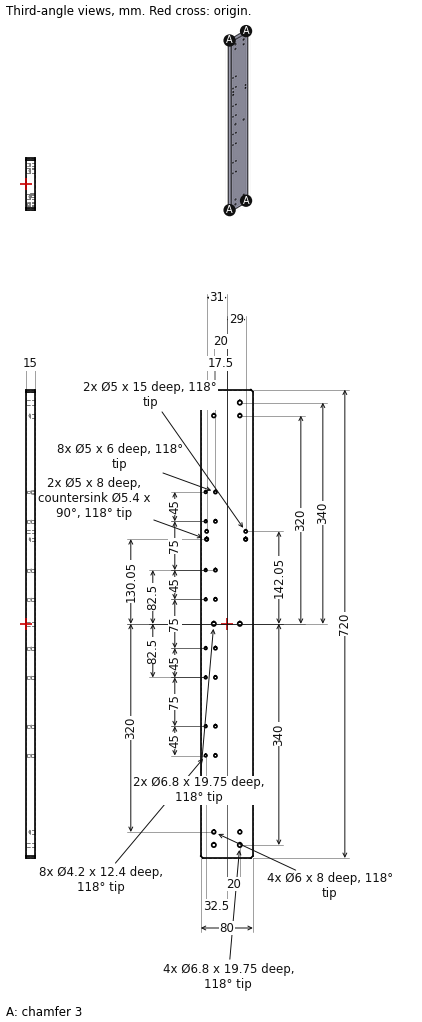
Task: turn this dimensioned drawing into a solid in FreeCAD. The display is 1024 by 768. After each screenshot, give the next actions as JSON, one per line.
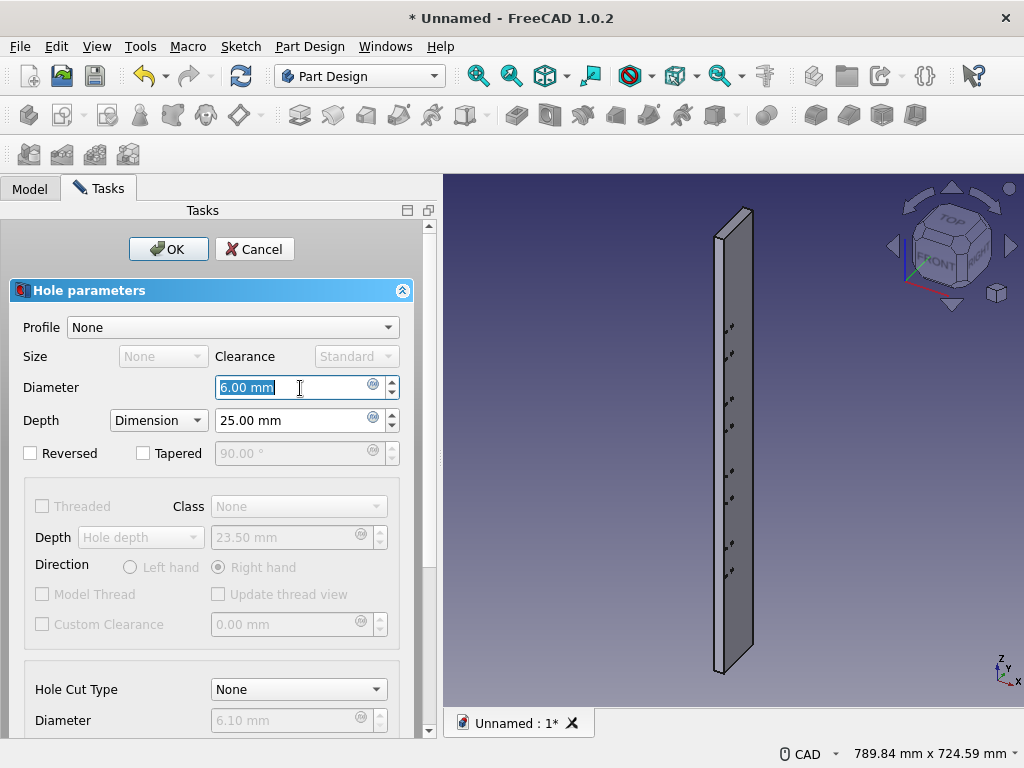
{"action": "type", "text": "5"}
{"action": "key", "text": "Tab"}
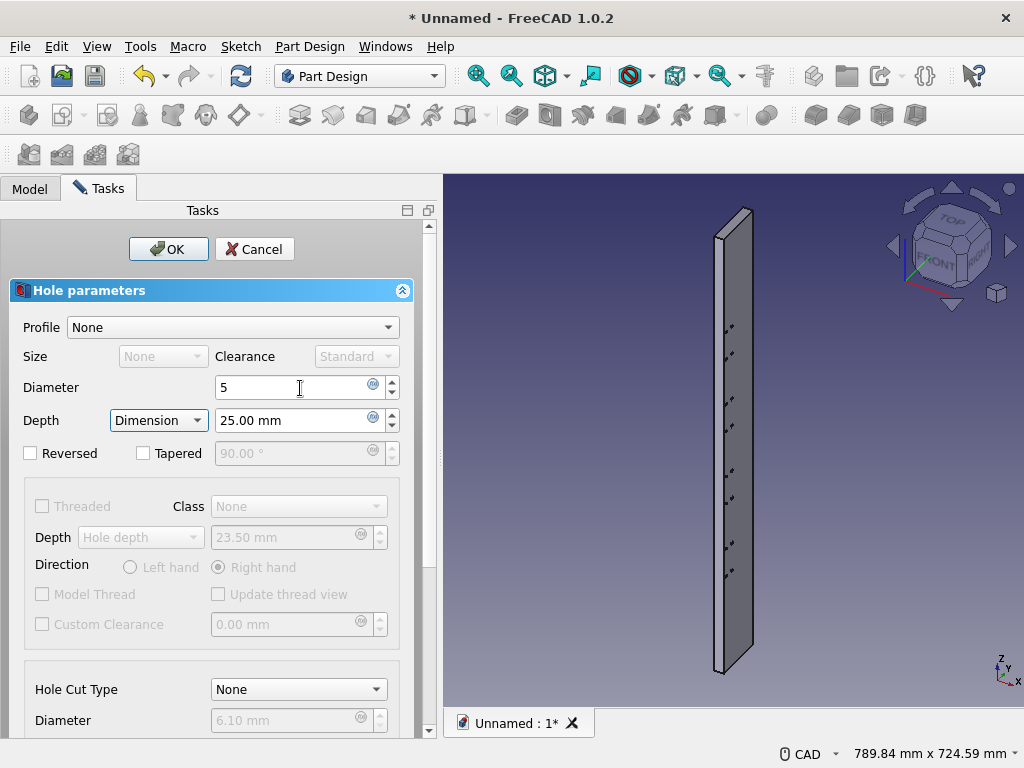
{"action": "triple_click", "coordinate": [300, 420]}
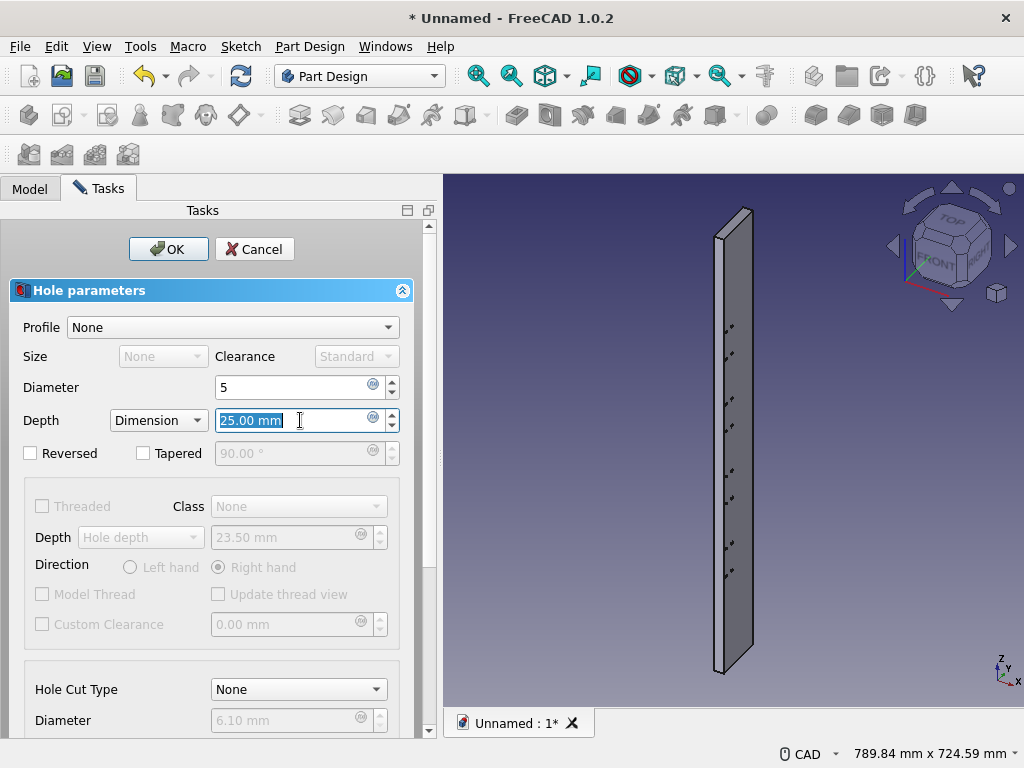
{"action": "type", "text": "6"}
{"action": "key", "text": "Tab"}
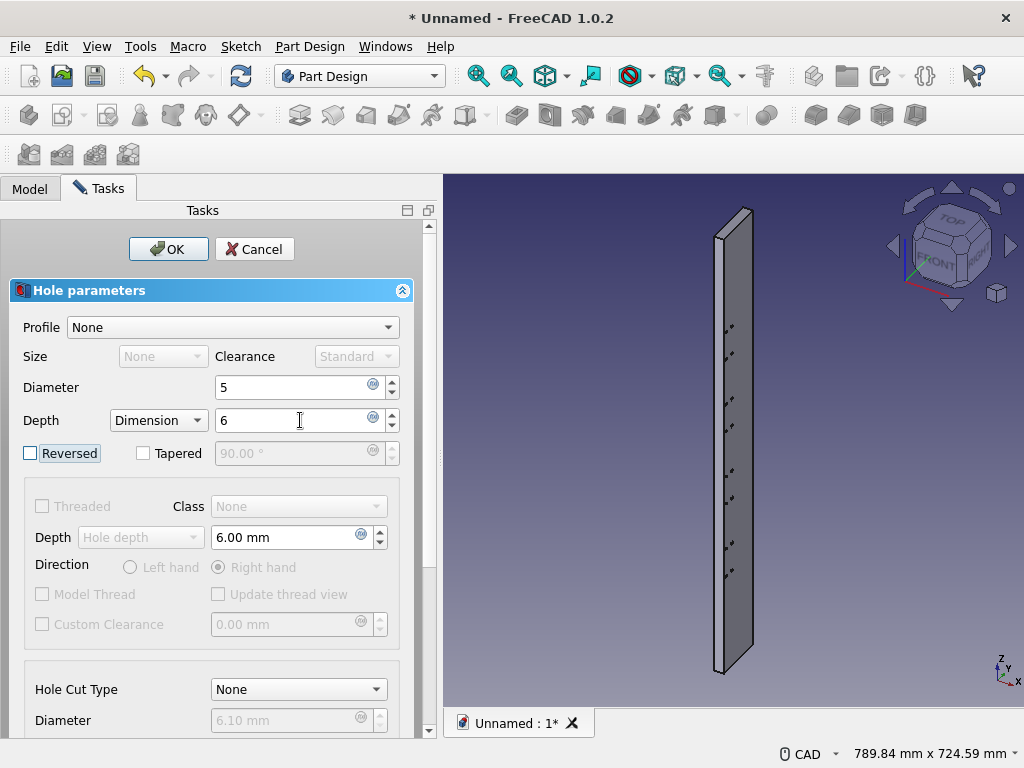
{"action": "left_click", "coordinate": [169, 249]}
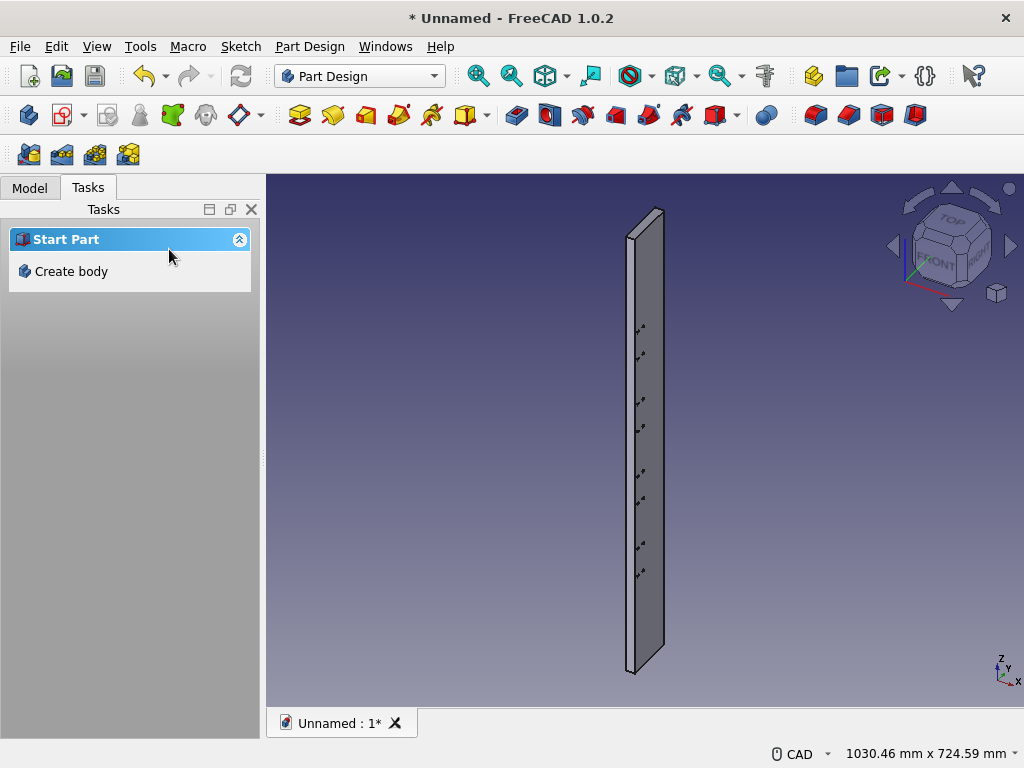
{"action": "left_click", "coordinate": [650, 627]}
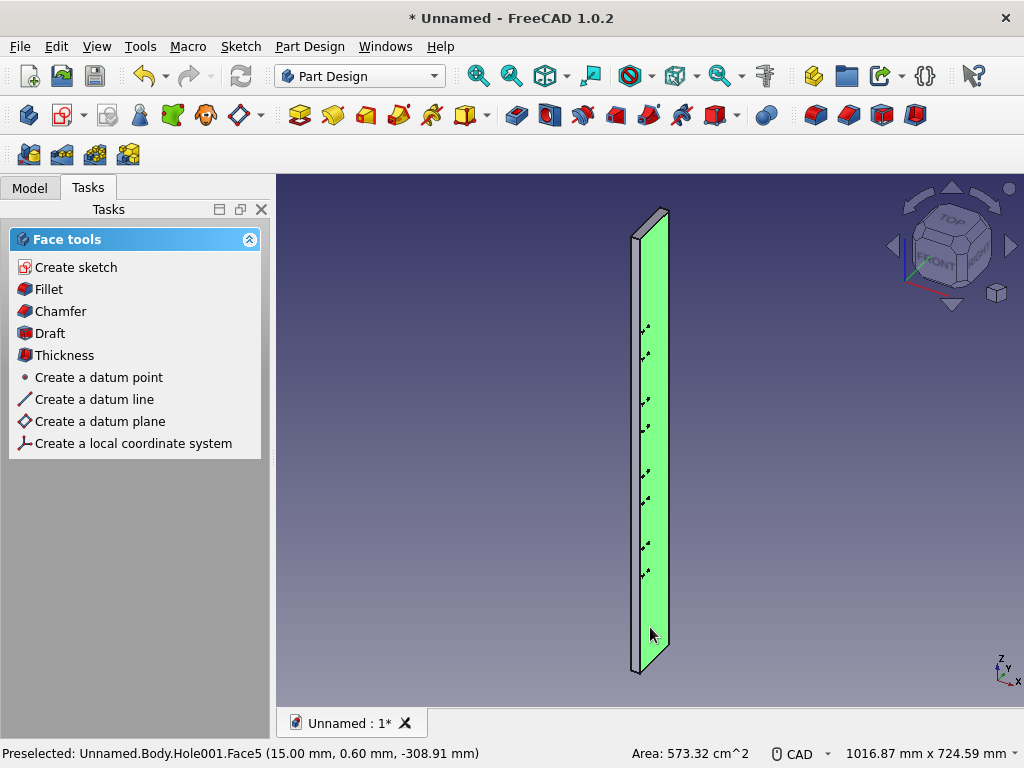
{"action": "left_click", "coordinate": [62, 116]}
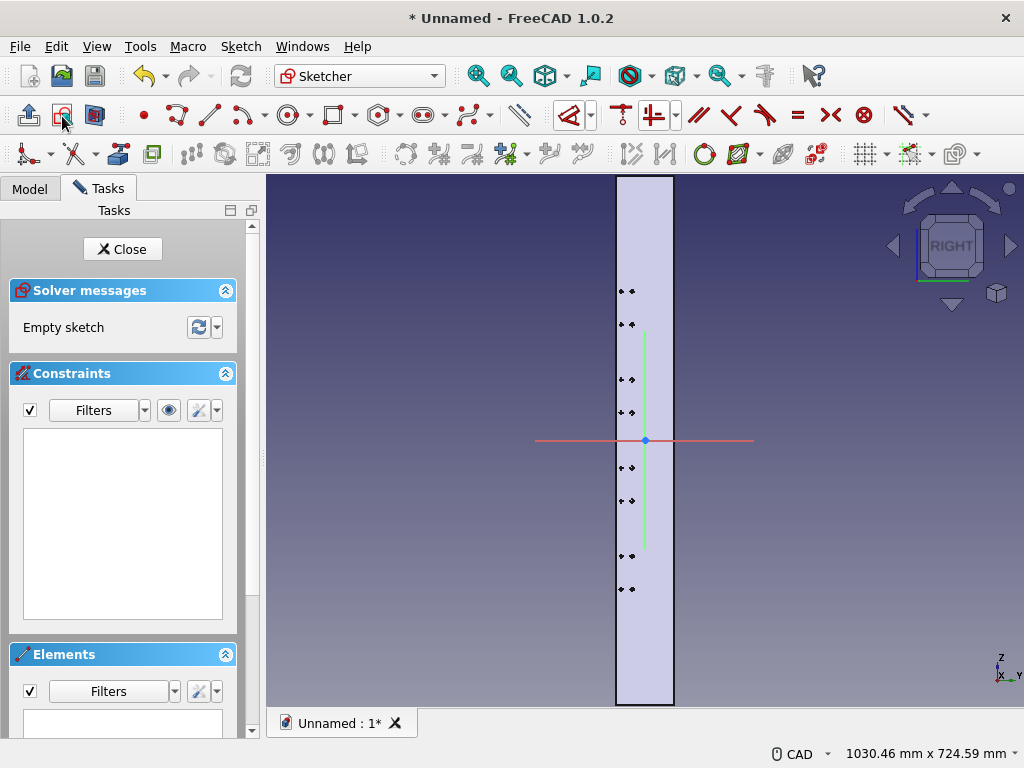
{"action": "scroll", "coordinate": [437, 440], "scroll_direction": "down", "scroll_amount": 2}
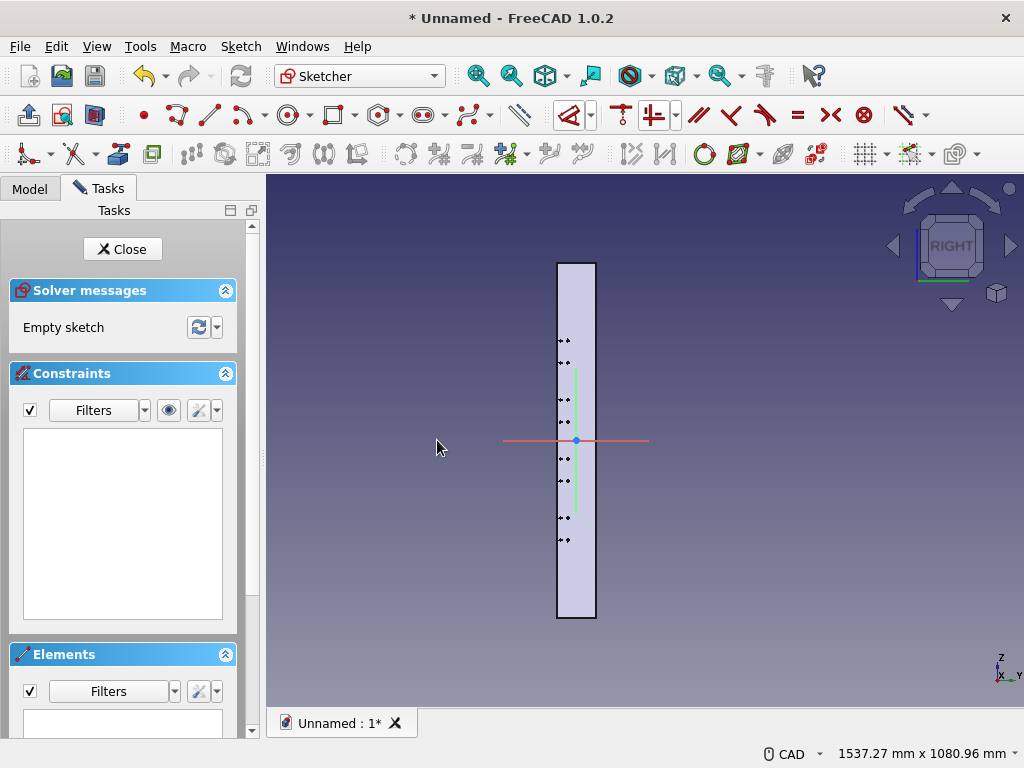
{"action": "left_click", "coordinate": [288, 116]}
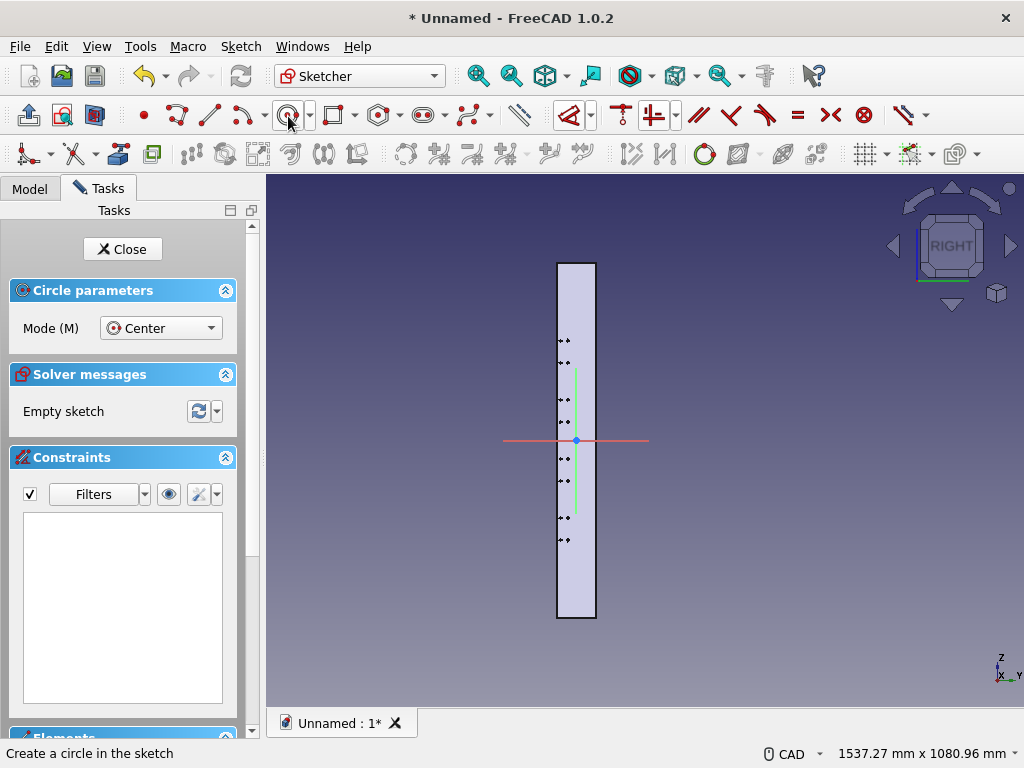
{"action": "scroll", "coordinate": [586, 608], "scroll_direction": "up", "scroll_amount": 14}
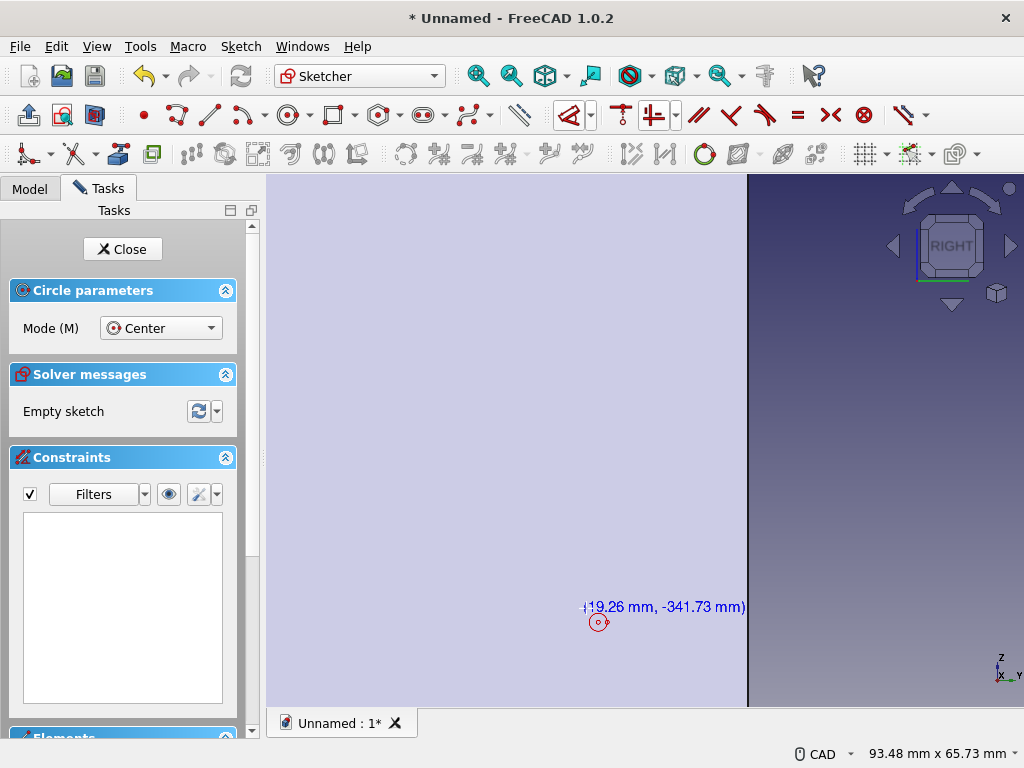
{"action": "scroll", "coordinate": [586, 609], "scroll_direction": "down", "scroll_amount": 14}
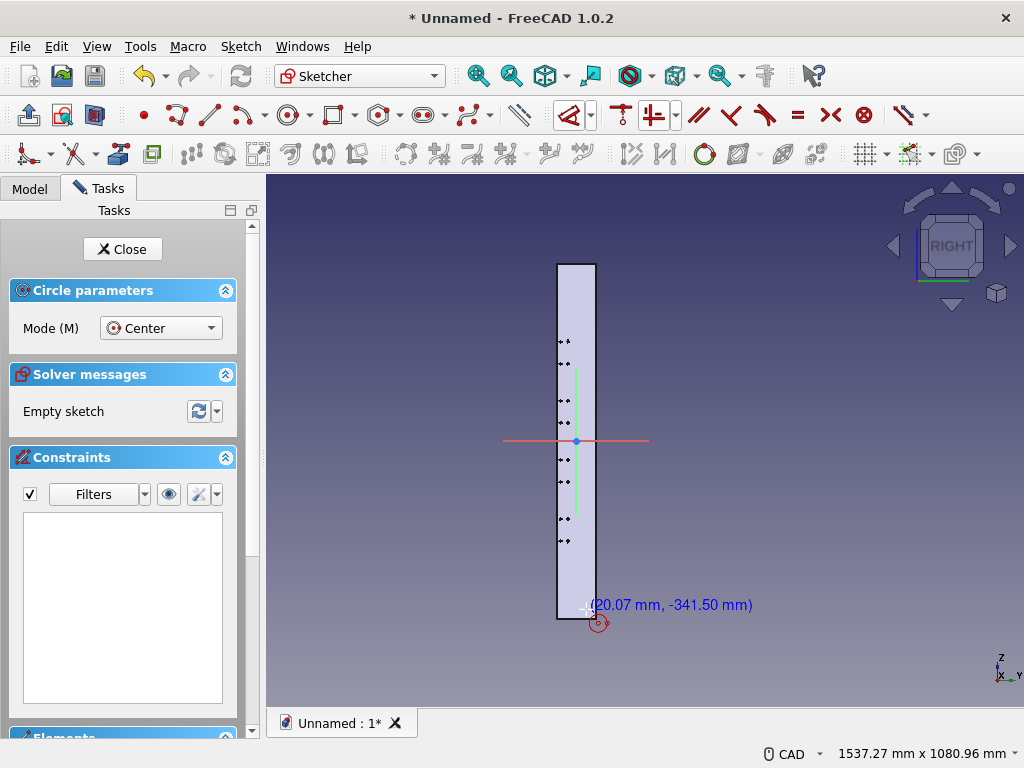
{"action": "scroll", "coordinate": [586, 609], "scroll_direction": "up", "scroll_amount": 3}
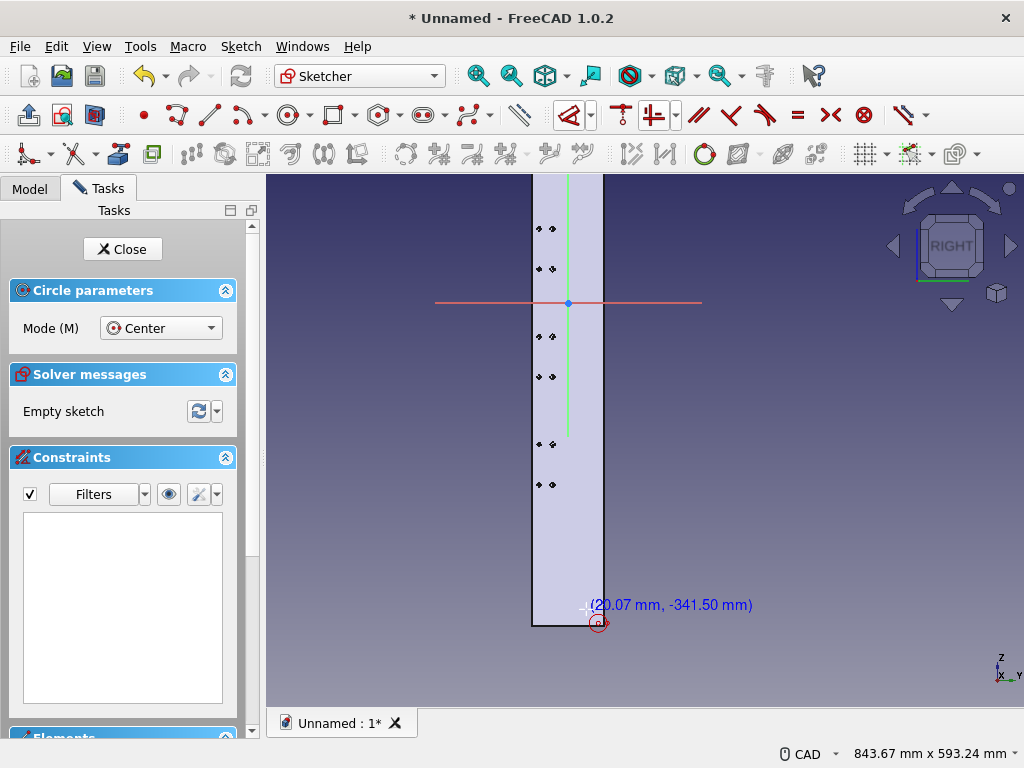
{"action": "left_click", "coordinate": [586, 608]}
{"action": "mouse_move", "coordinate": [588, 606]}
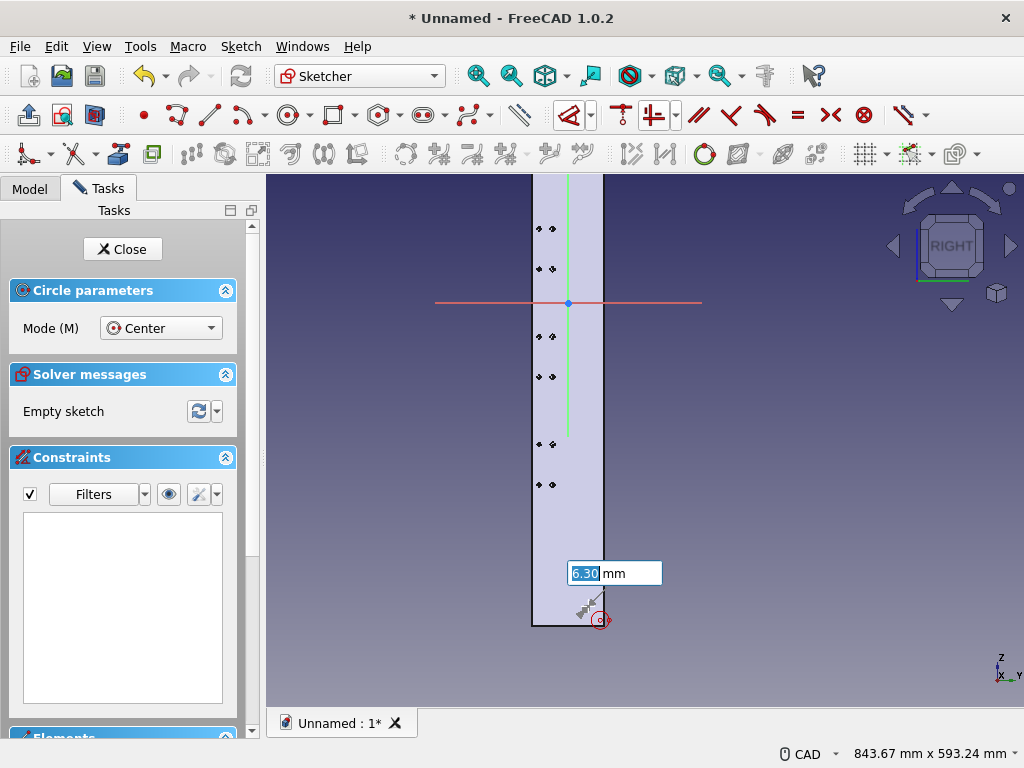
{"action": "type", "text": "6.8"}
{"action": "key", "text": "Return"}